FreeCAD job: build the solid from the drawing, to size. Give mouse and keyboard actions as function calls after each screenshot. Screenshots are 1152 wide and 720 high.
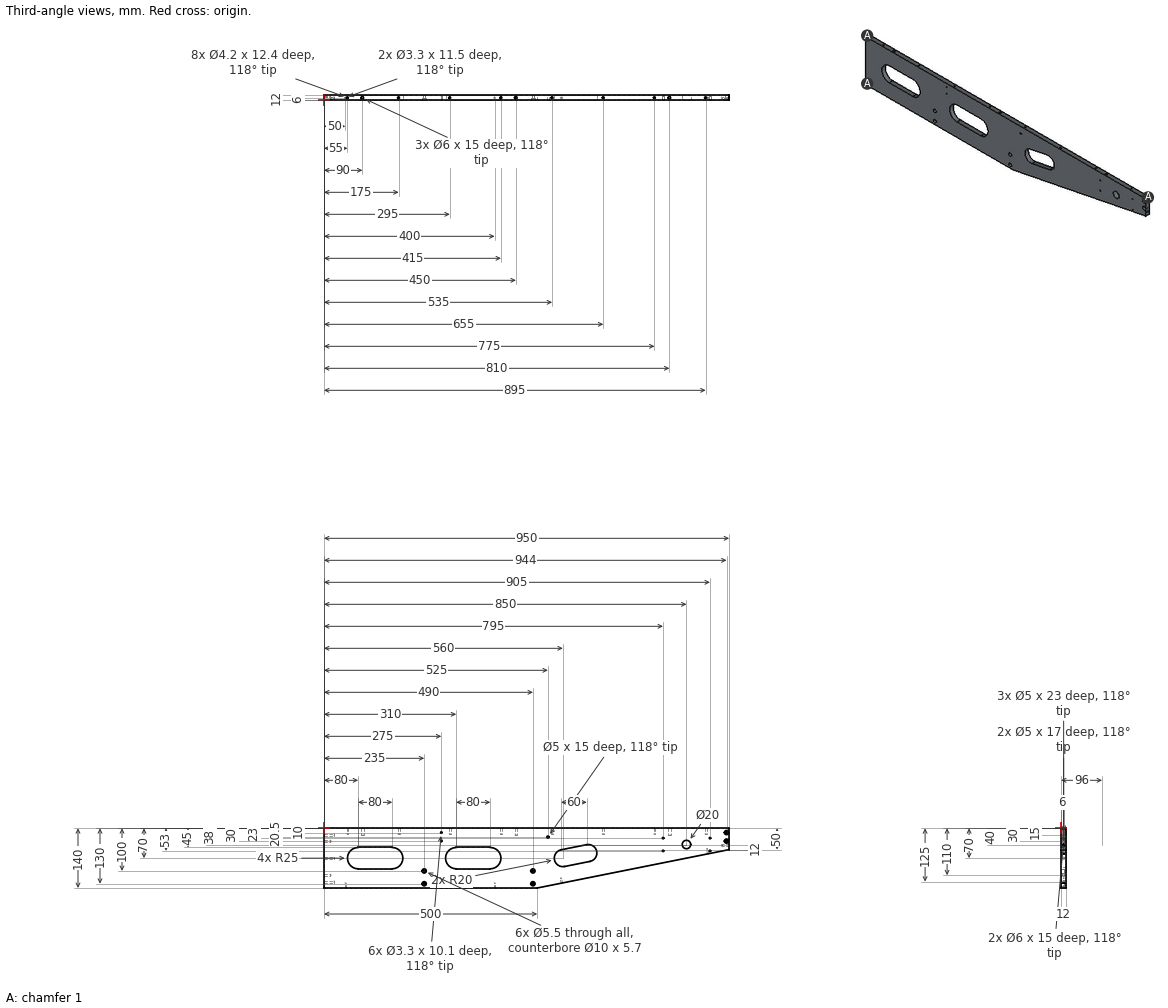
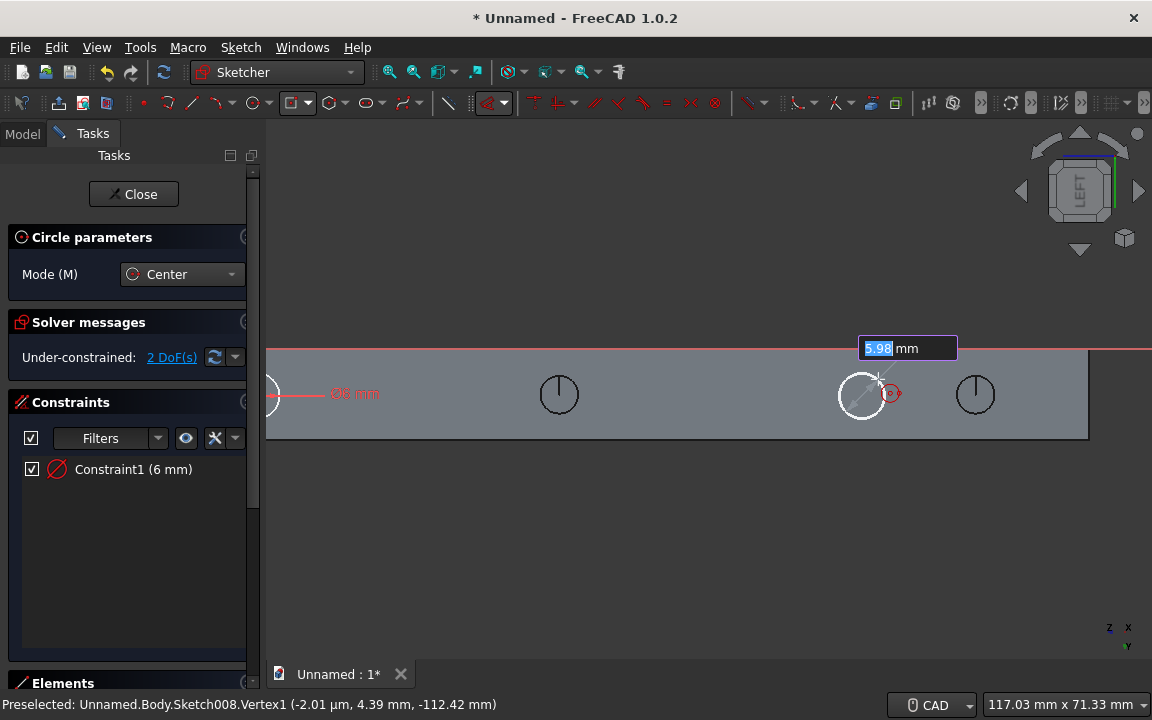
text(6)
key(Return)
key(Escape)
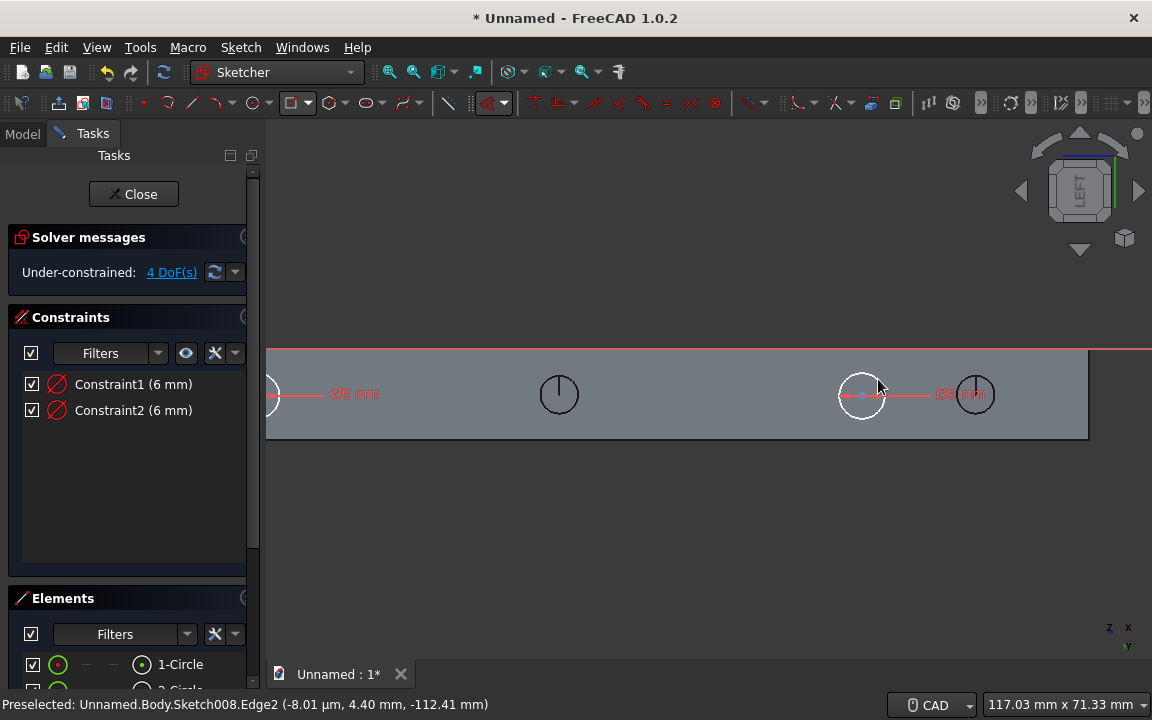
scroll(864, 396, down, 3)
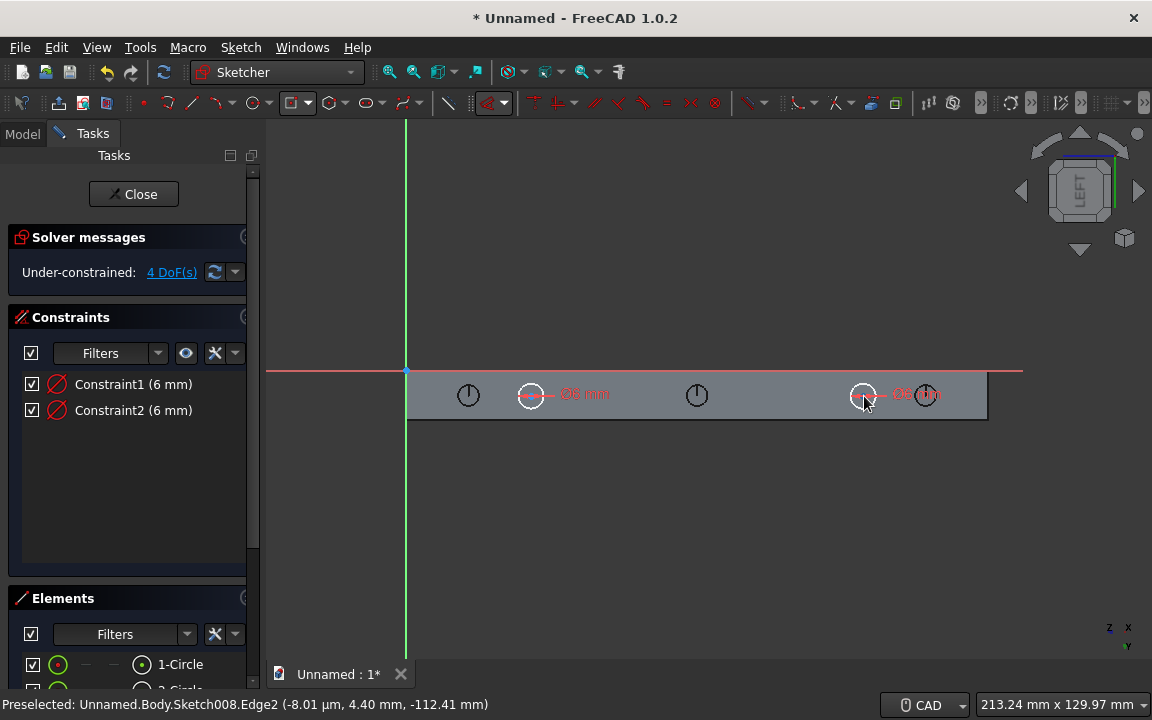
click(531, 396)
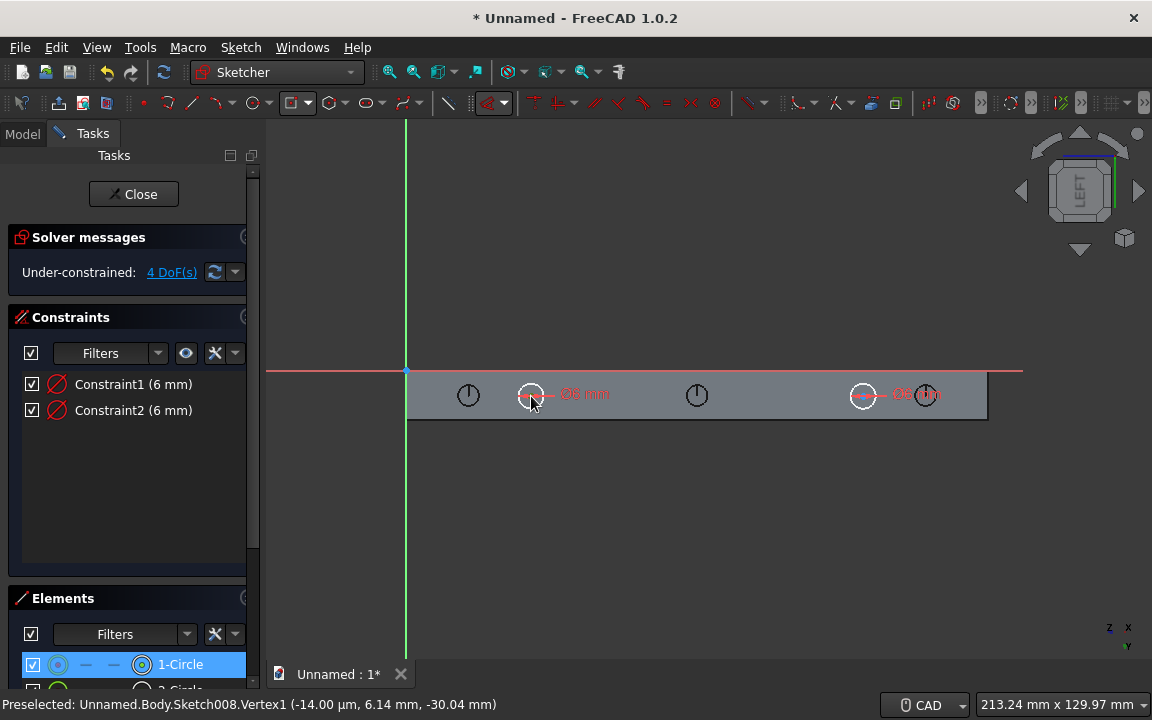
click(863, 396)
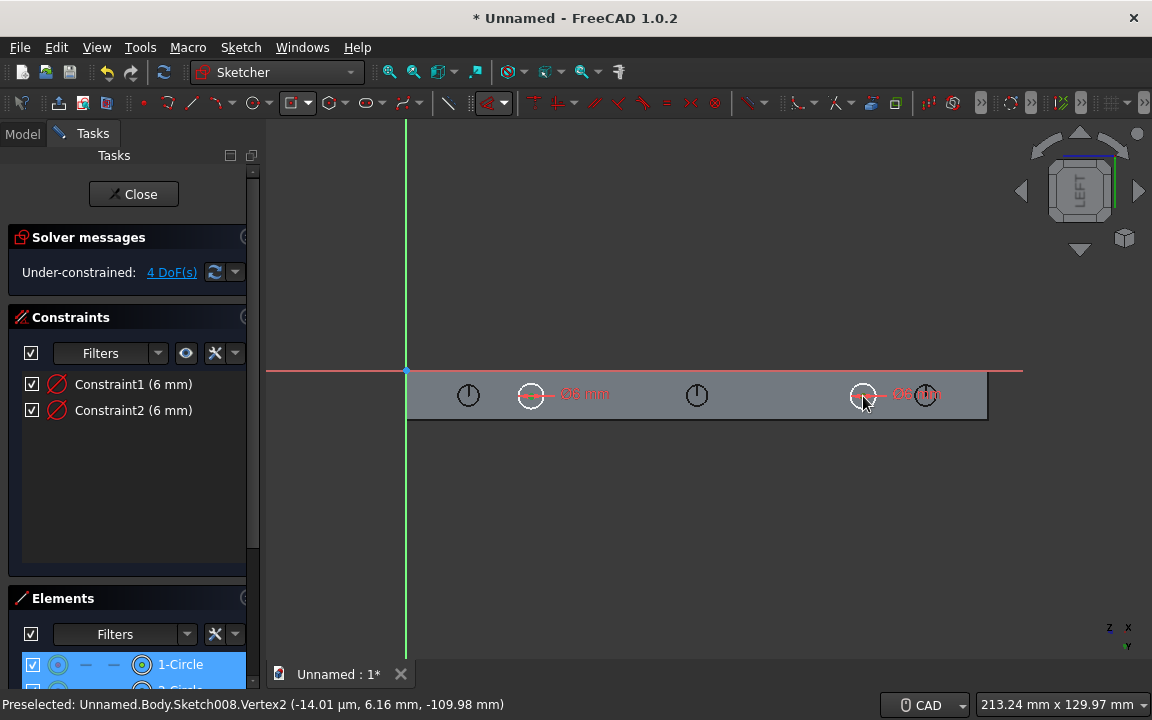
key(h)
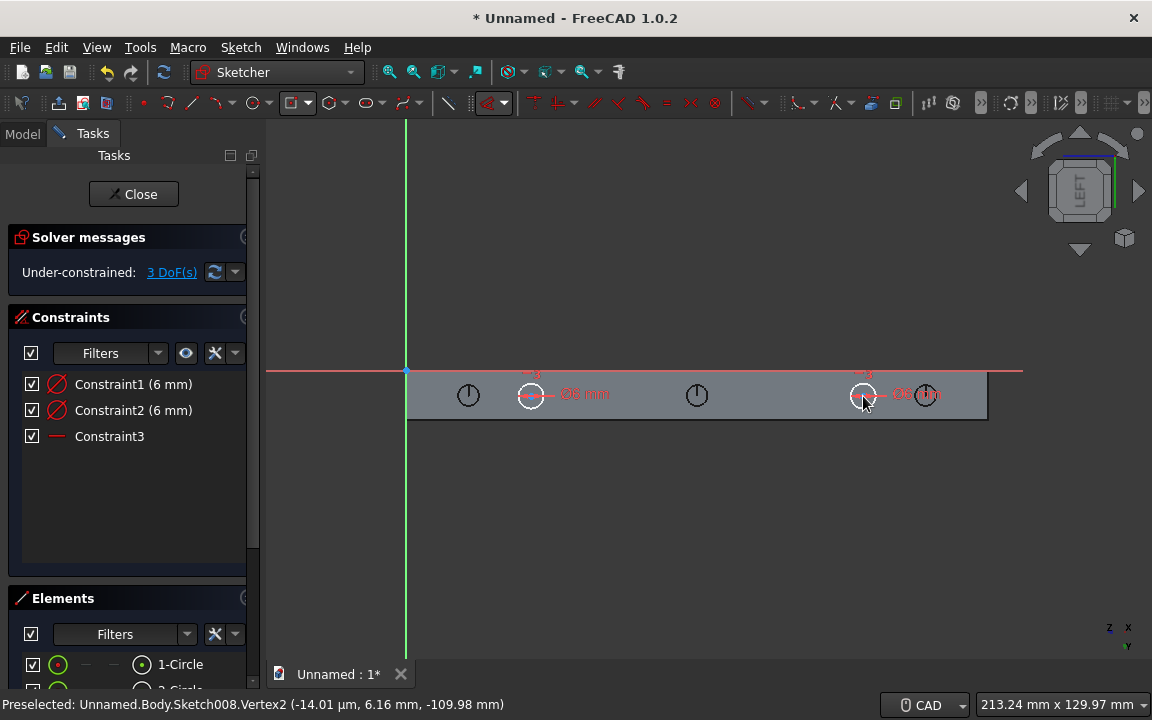
scroll(531, 396, up, 3)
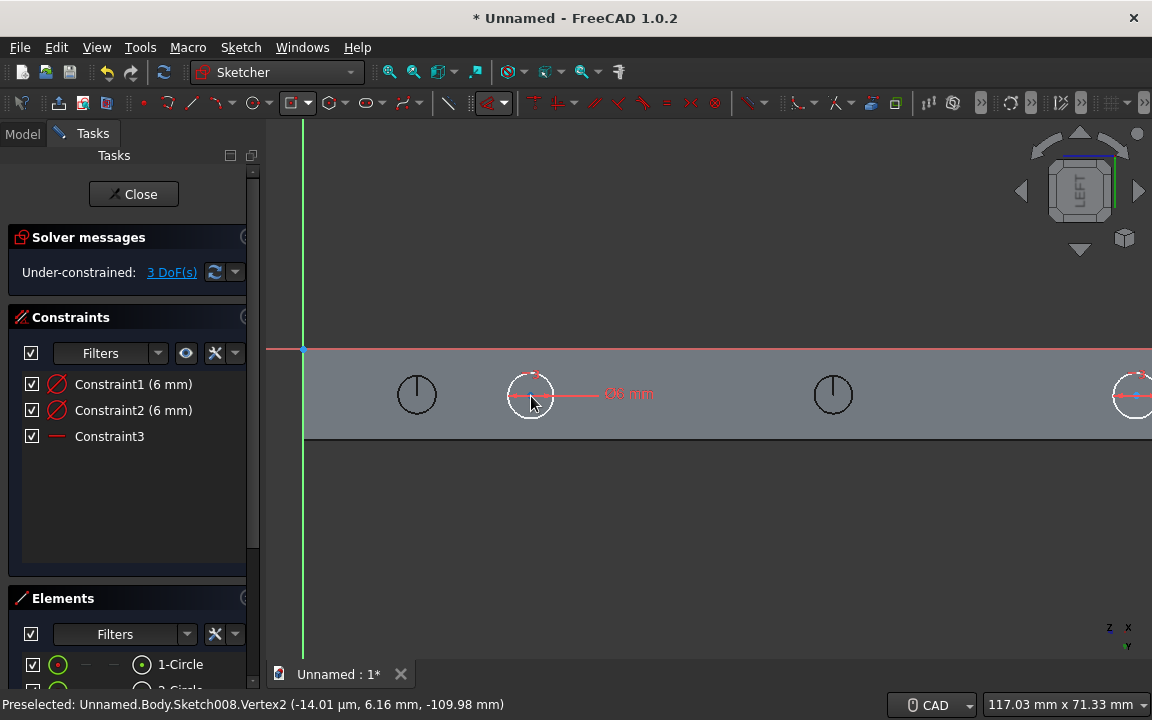
click(531, 396)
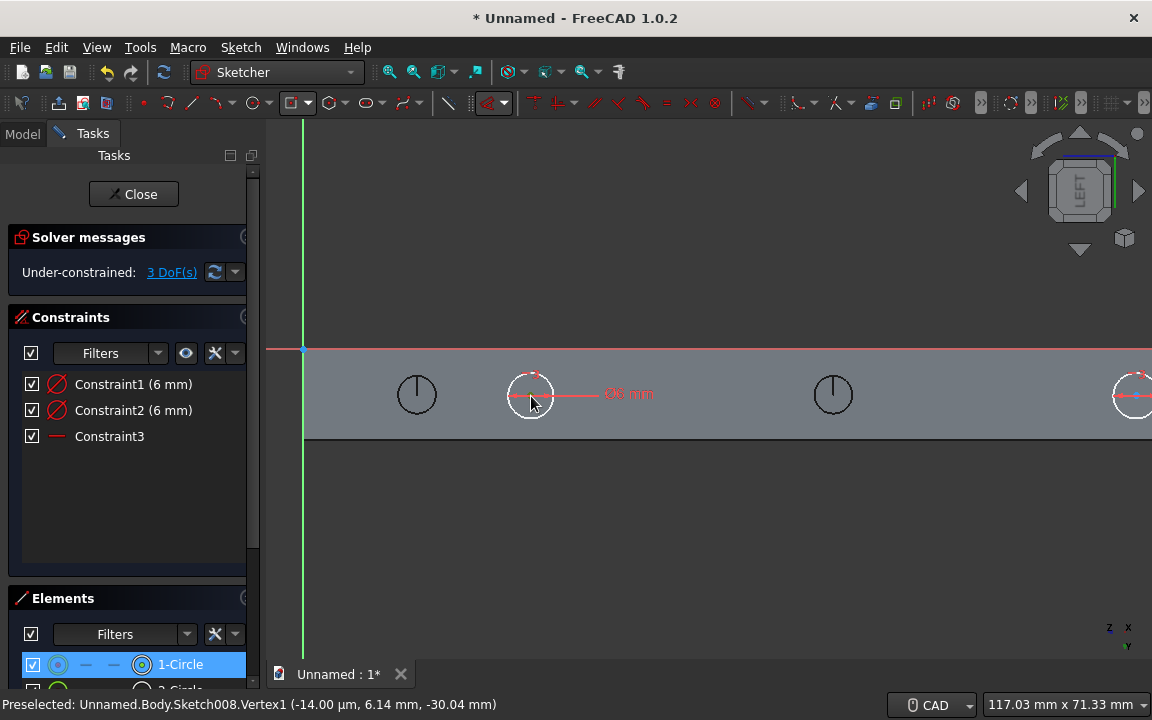
key(i)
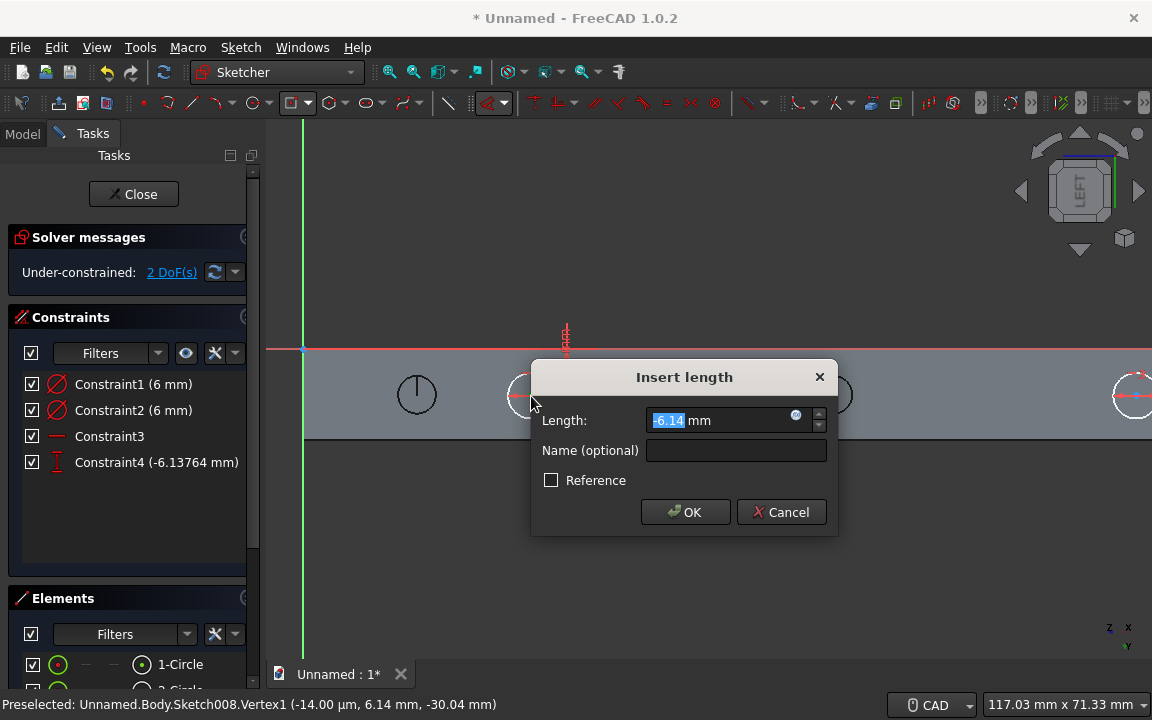
text(-6)
key(Return)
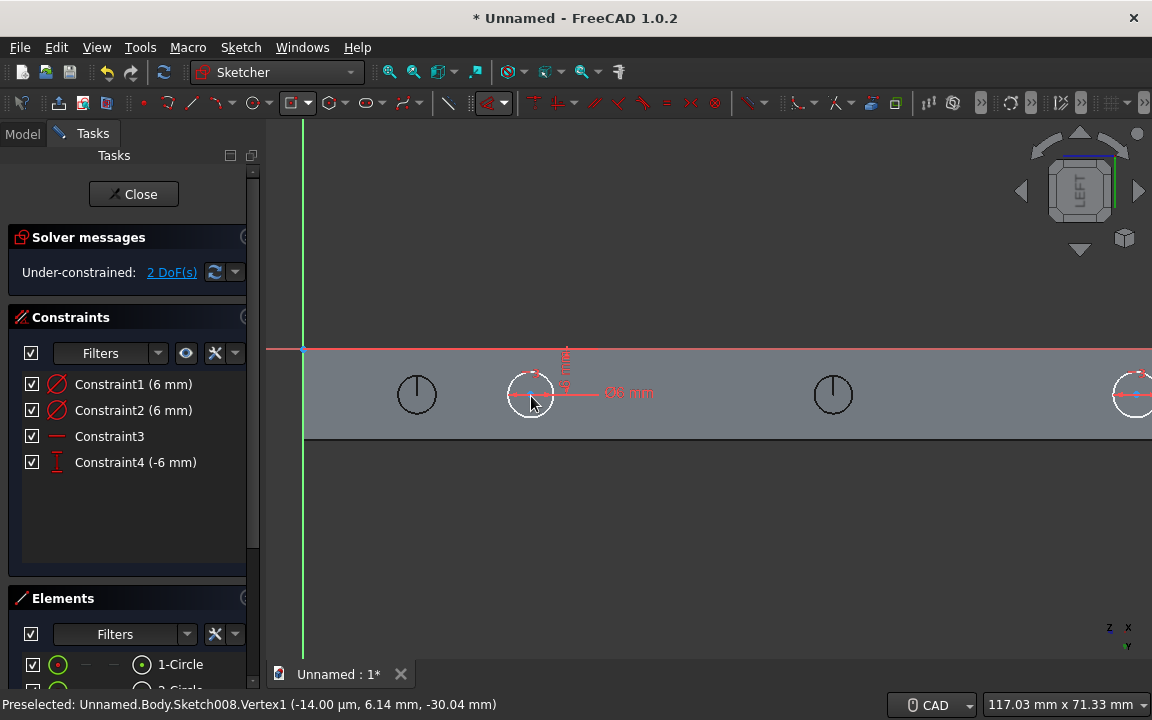
click(531, 395)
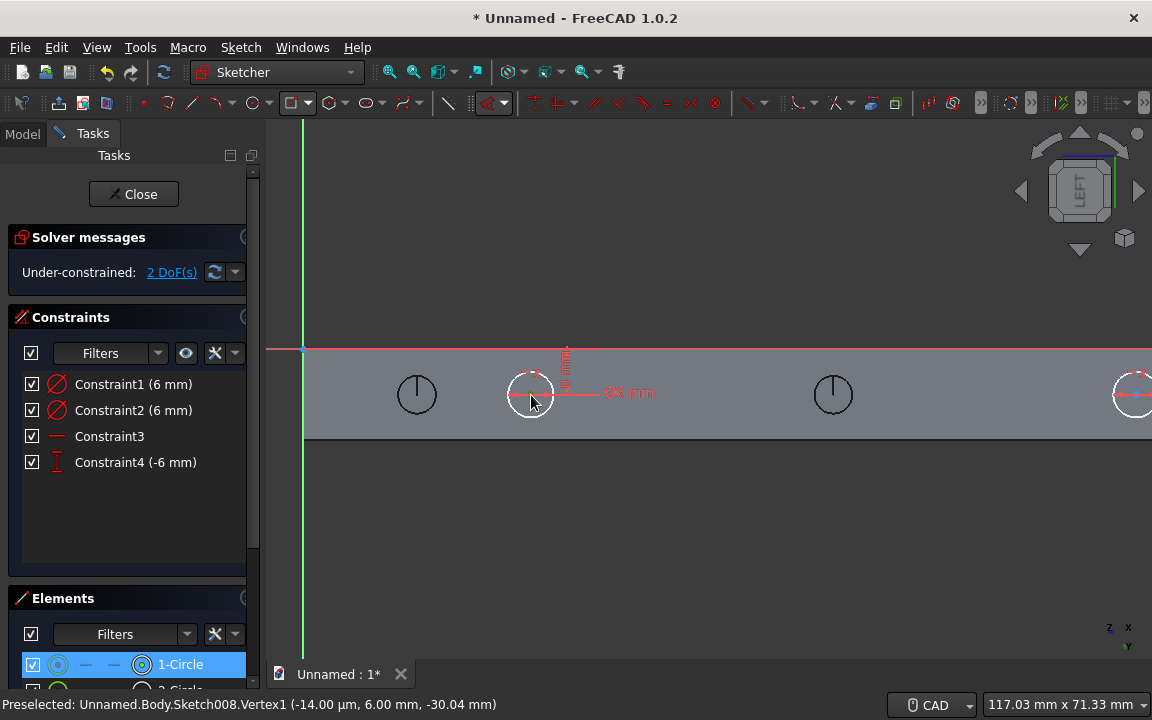
key(l)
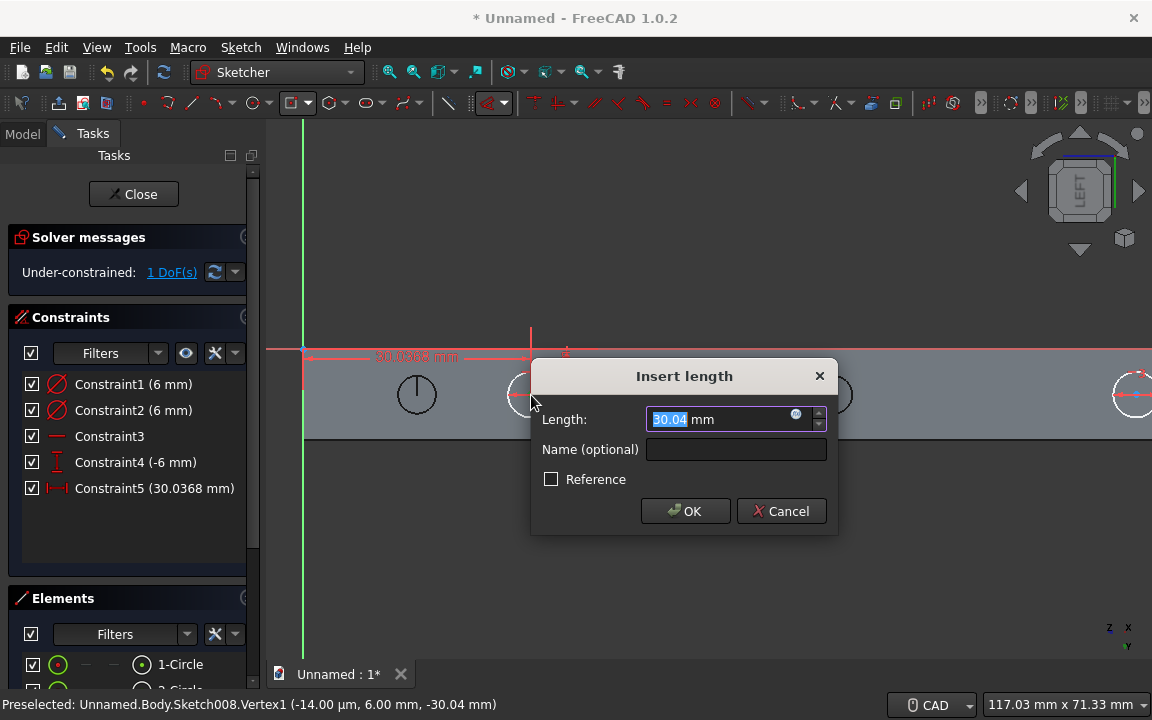
text(30)
key(Return)